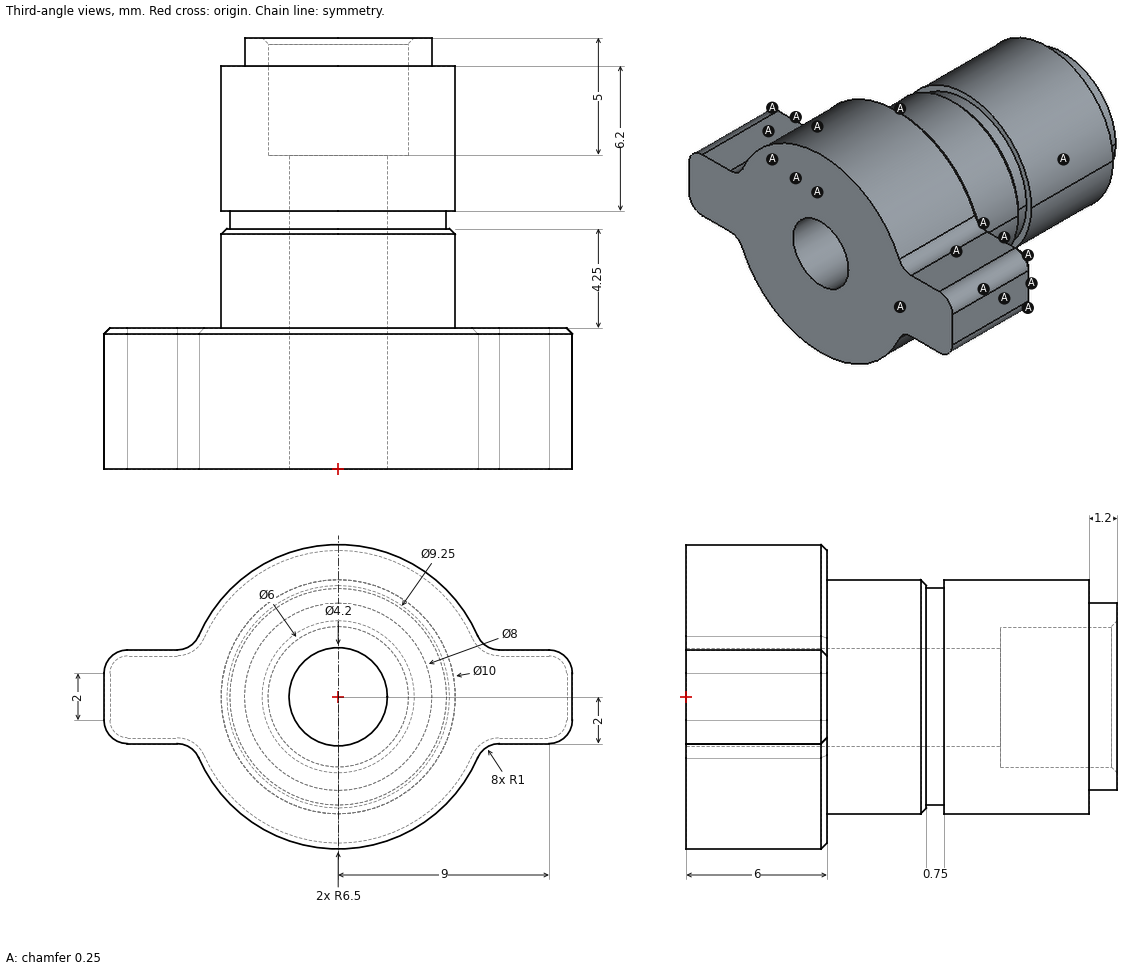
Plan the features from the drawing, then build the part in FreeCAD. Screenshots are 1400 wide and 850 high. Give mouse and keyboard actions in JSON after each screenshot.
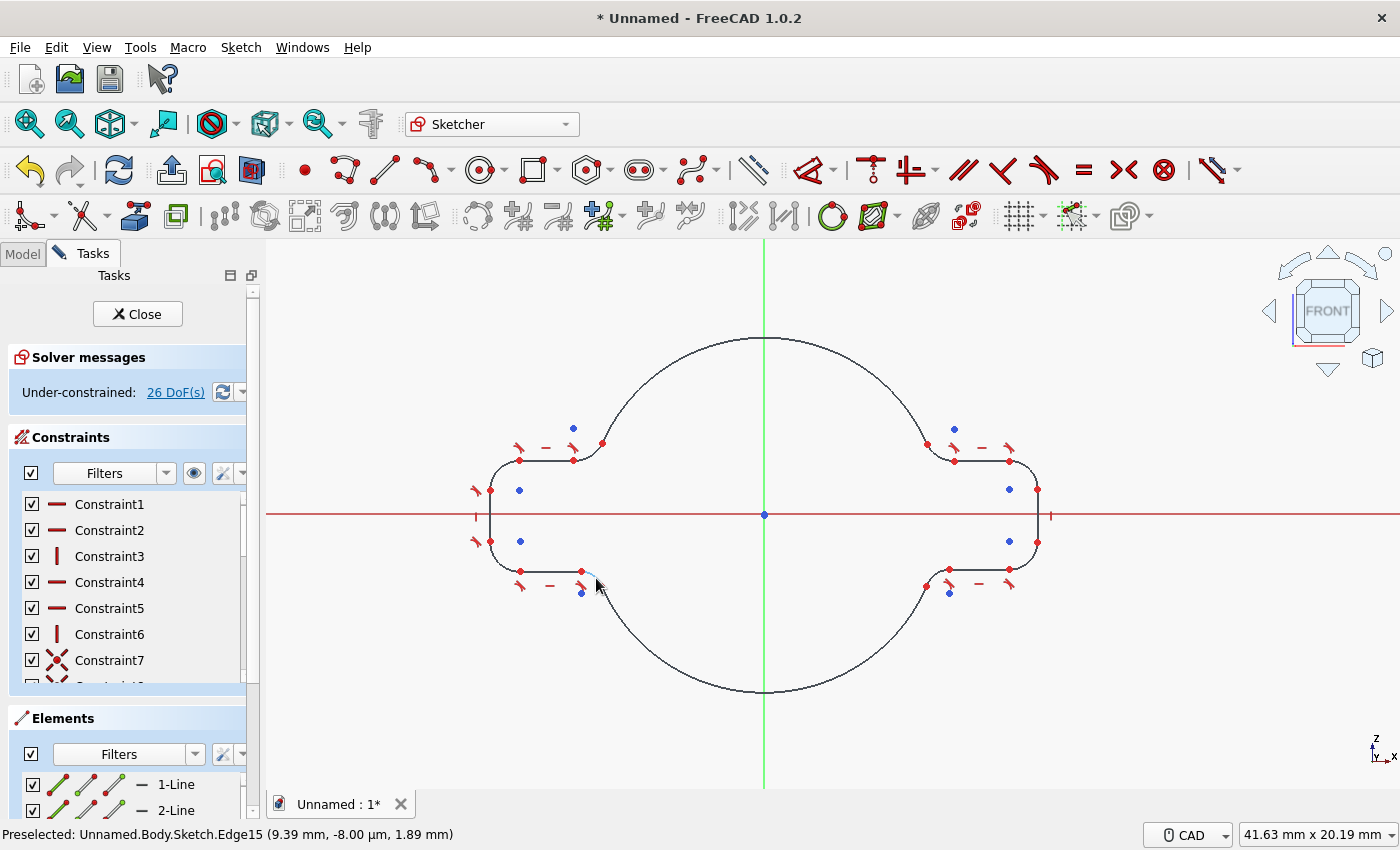
{"action": "scroll", "coordinate": [1038, 505], "scroll_direction": "up", "scroll_amount": 3}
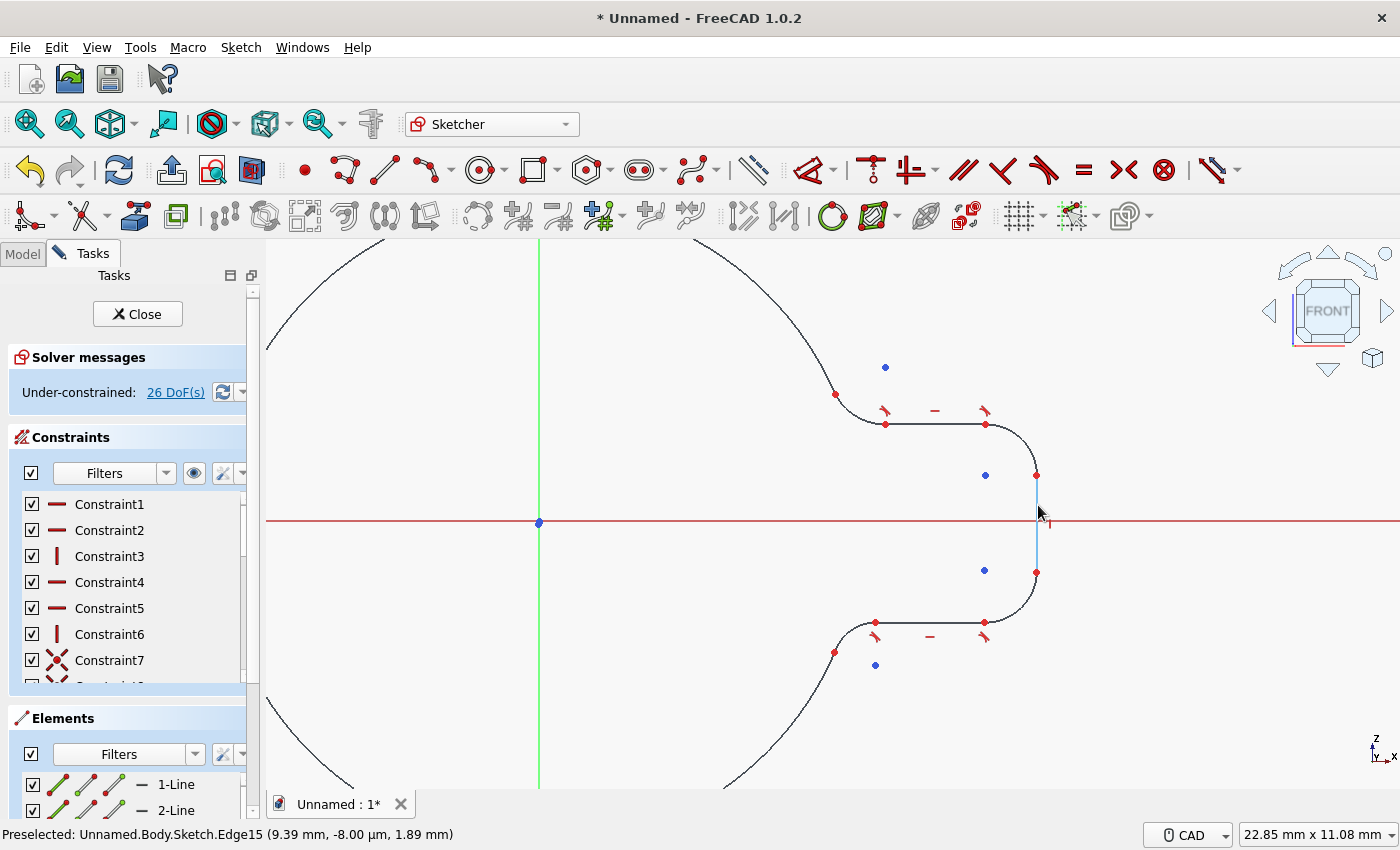
{"action": "left_click", "coordinate": [1037, 505]}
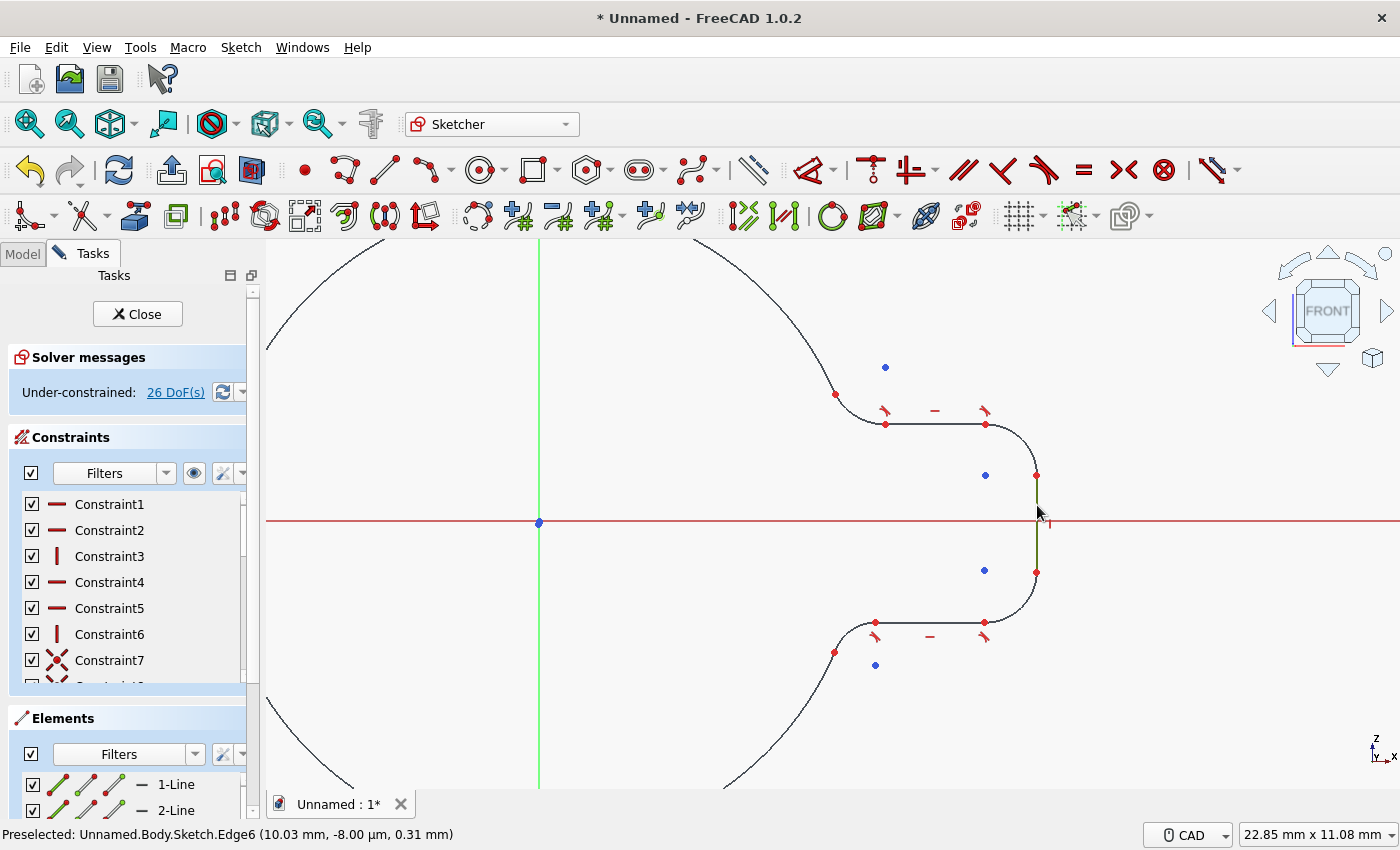
{"action": "left_click", "coordinate": [1031, 452]}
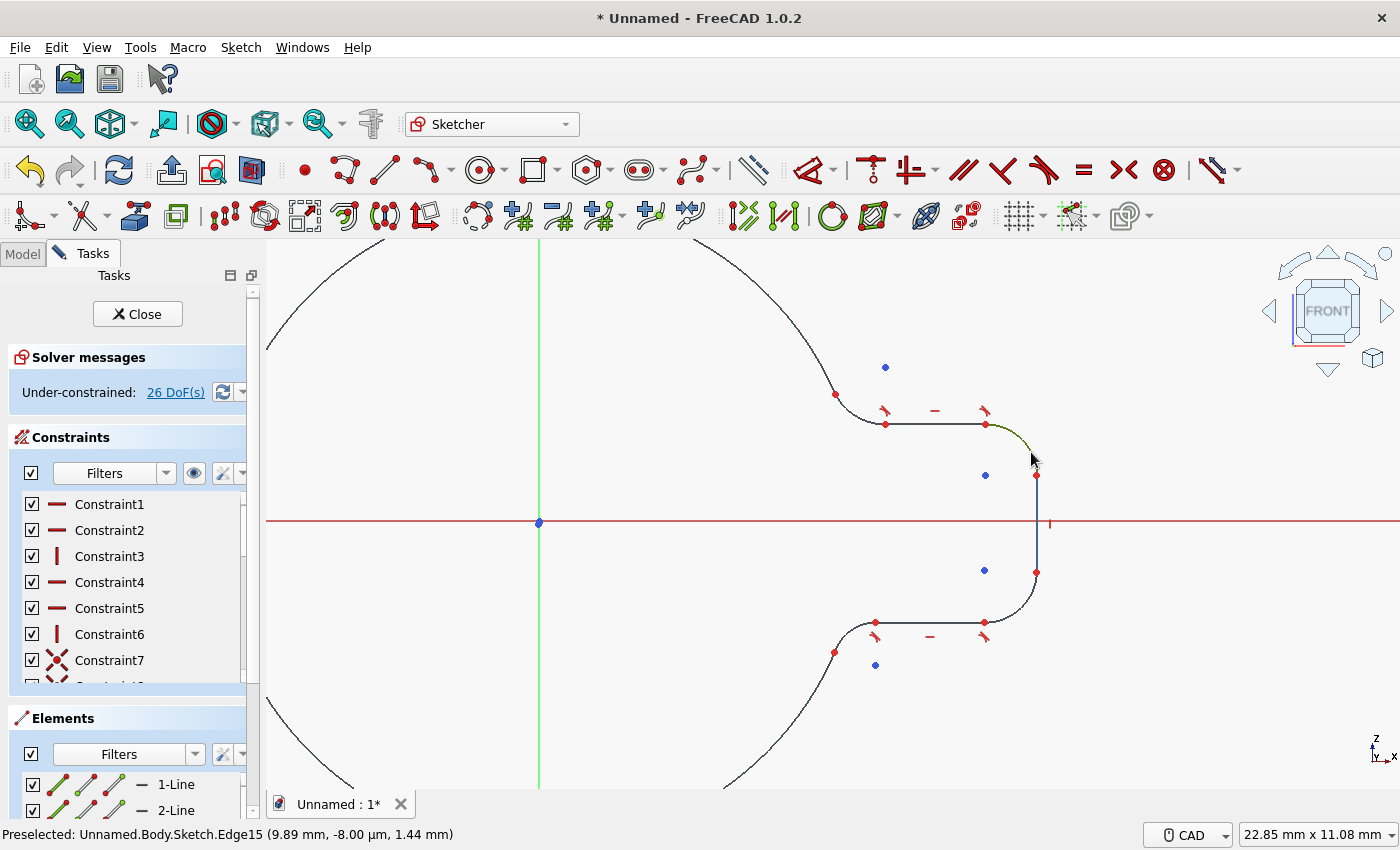
{"action": "left_click", "coordinate": [1044, 170]}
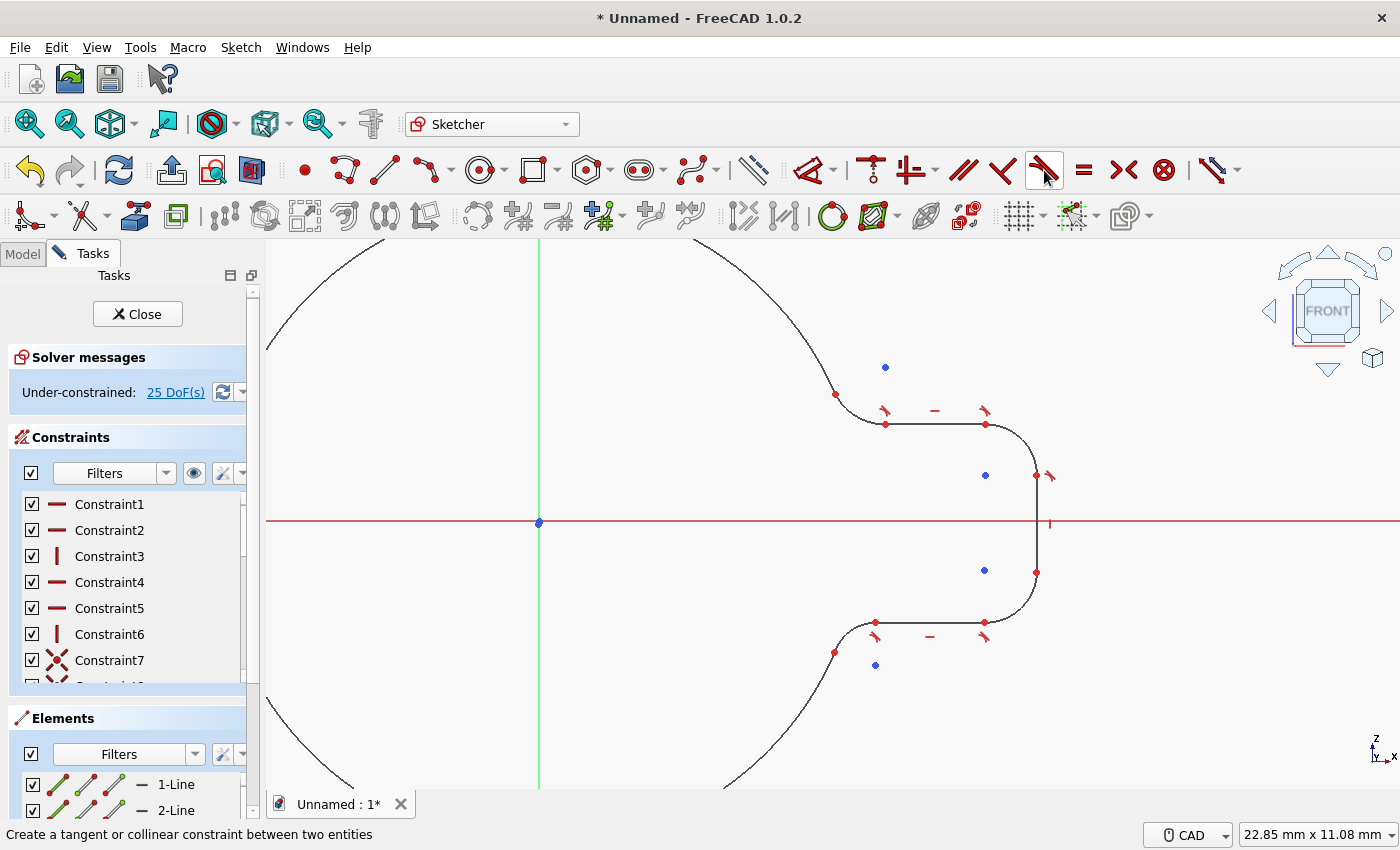
{"action": "left_click", "coordinate": [1037, 505]}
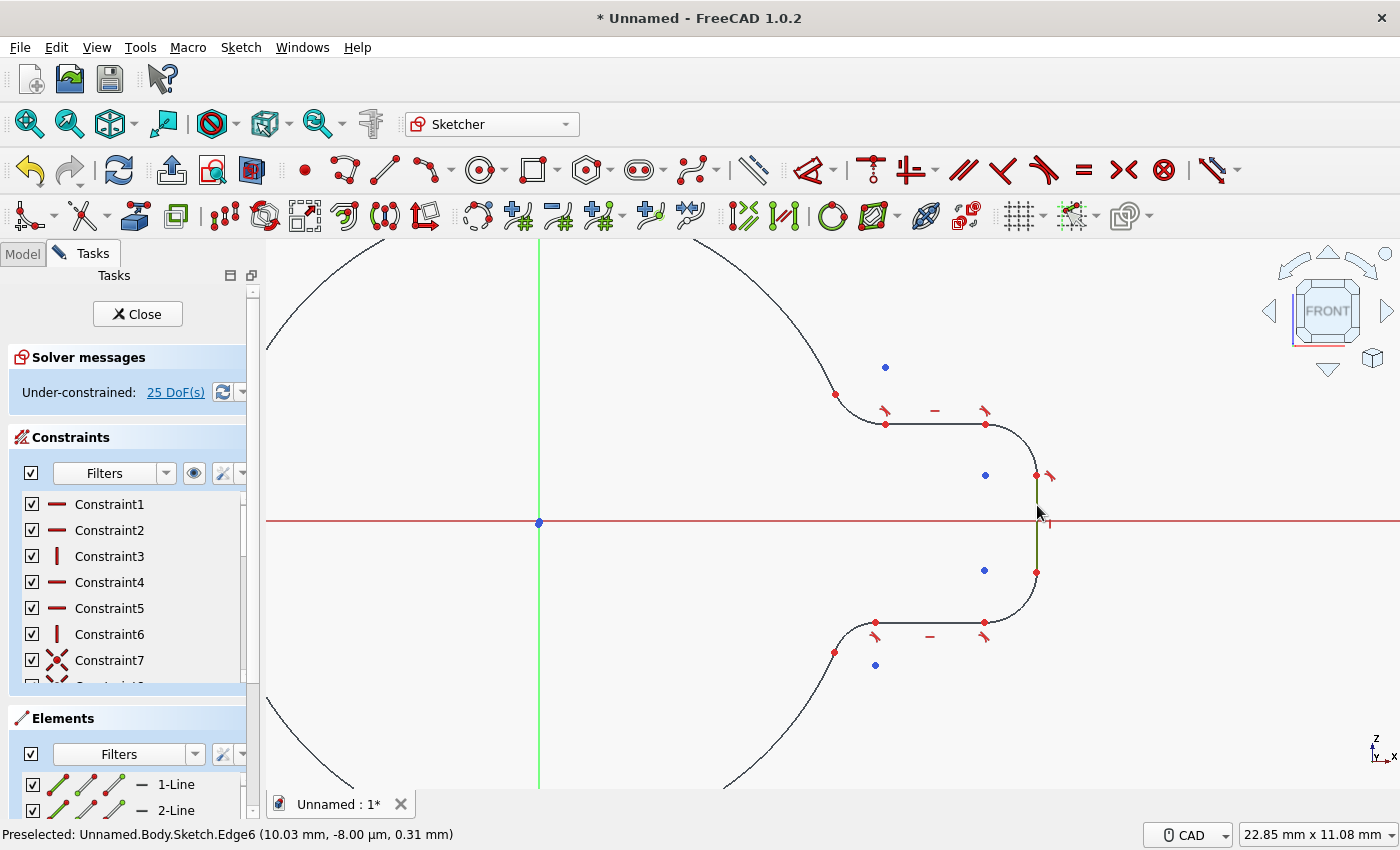
{"action": "left_click", "coordinate": [1008, 617]}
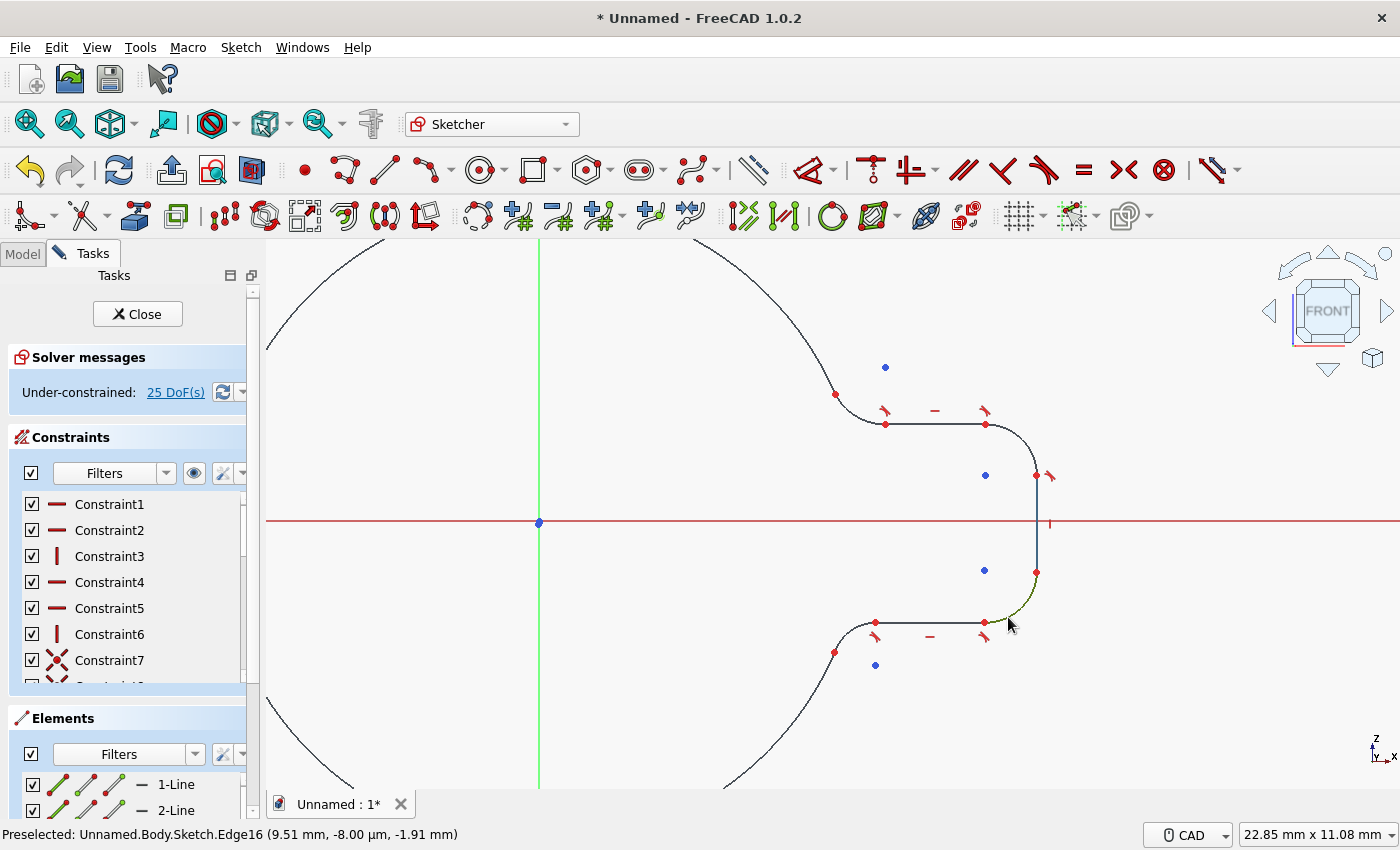
{"action": "left_click", "coordinate": [1044, 170]}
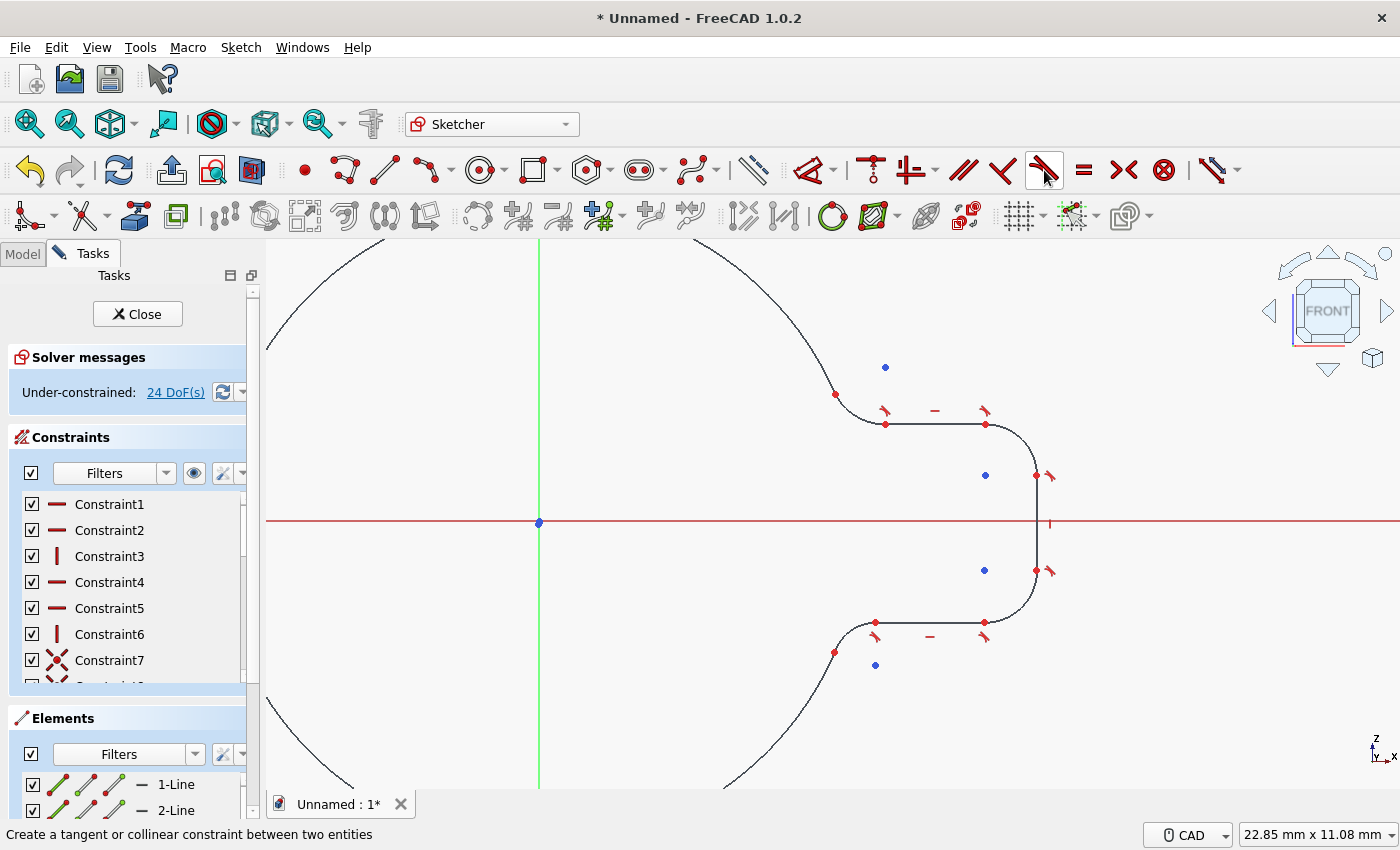
{"action": "left_click", "coordinate": [860, 626]}